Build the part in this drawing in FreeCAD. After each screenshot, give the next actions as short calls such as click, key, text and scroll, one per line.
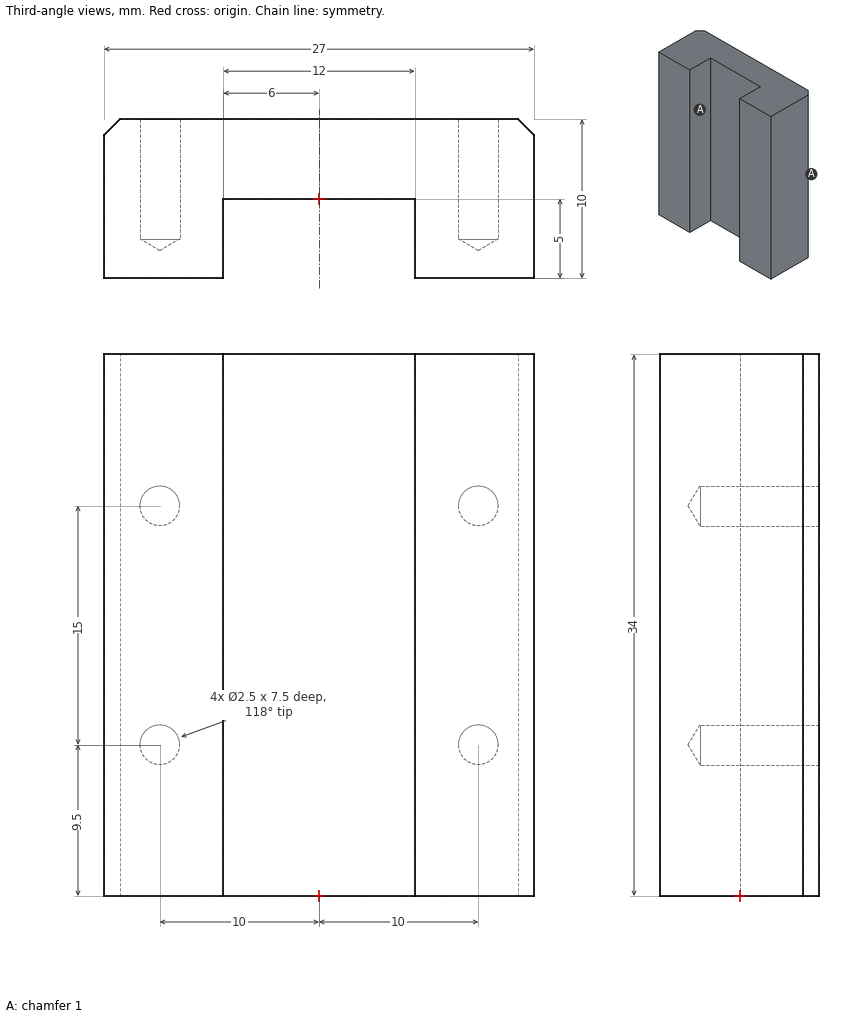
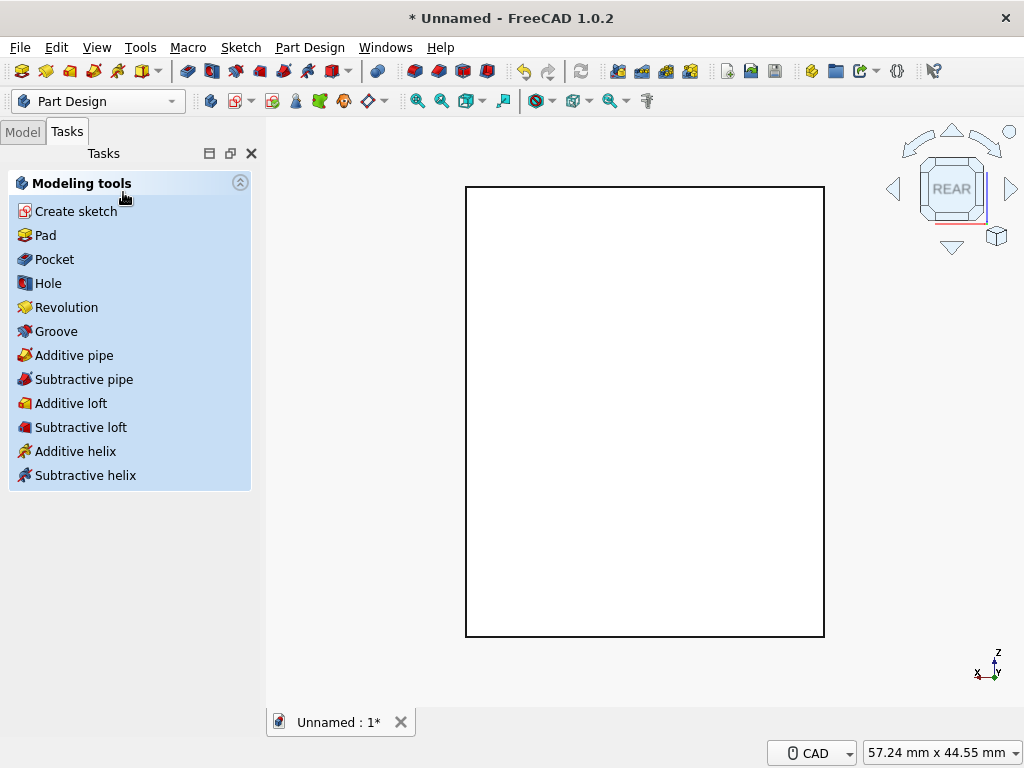
click(212, 72)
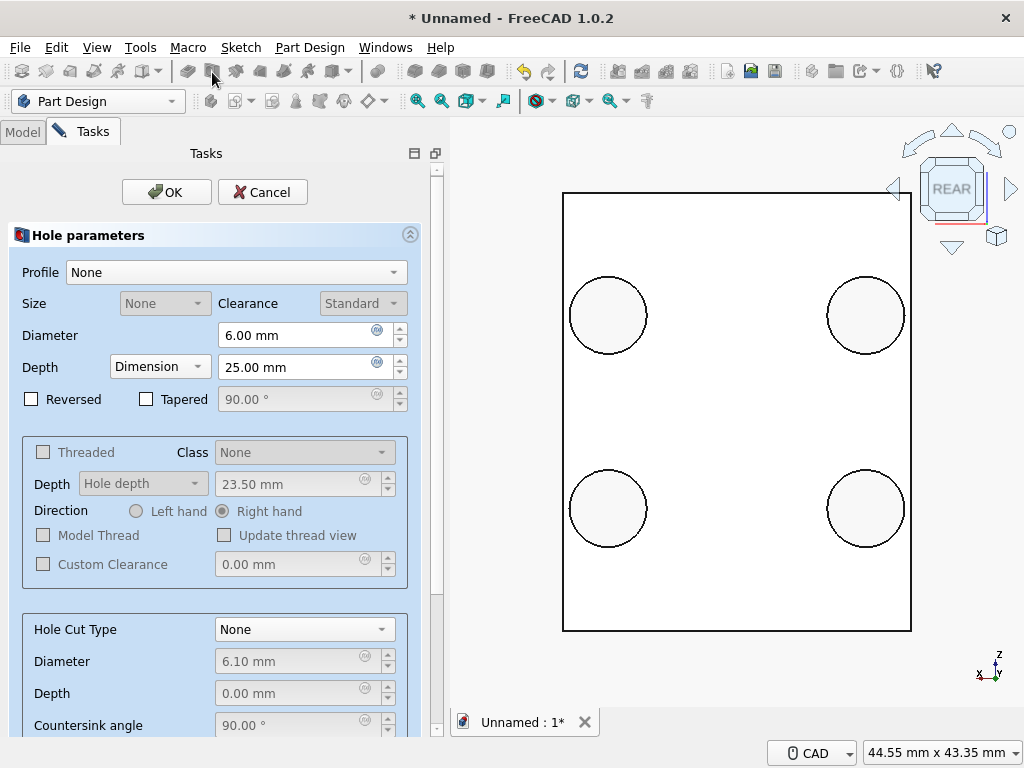
triple_click(305, 335)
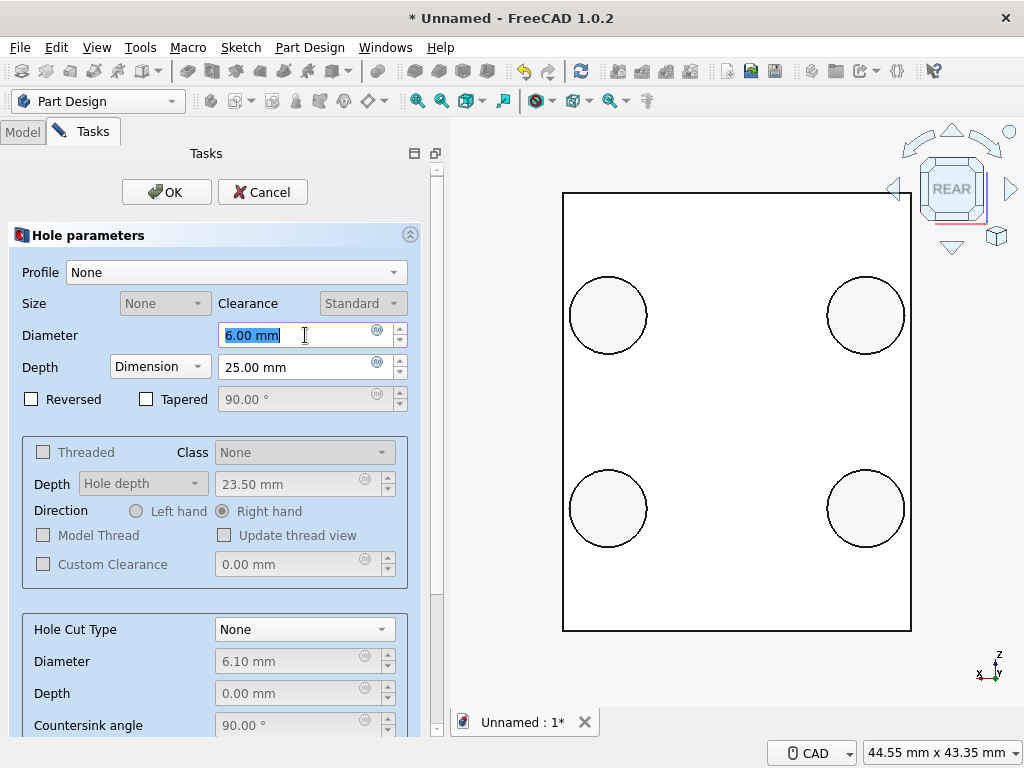
text(2.5)
key(Tab)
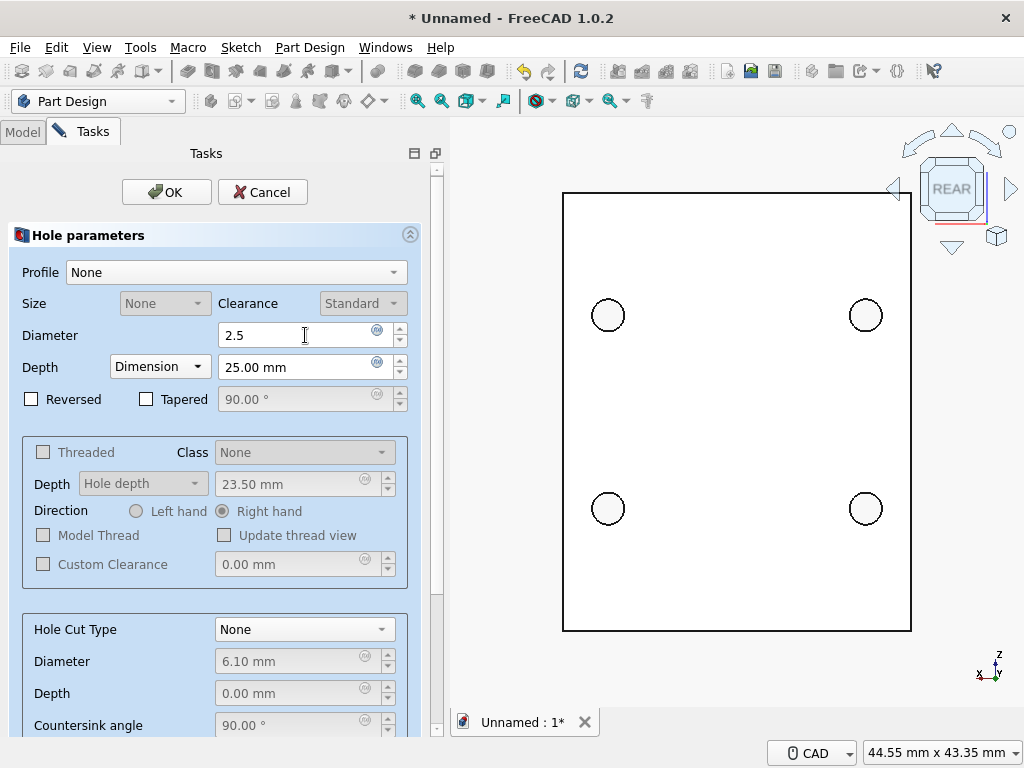
triple_click(305, 367)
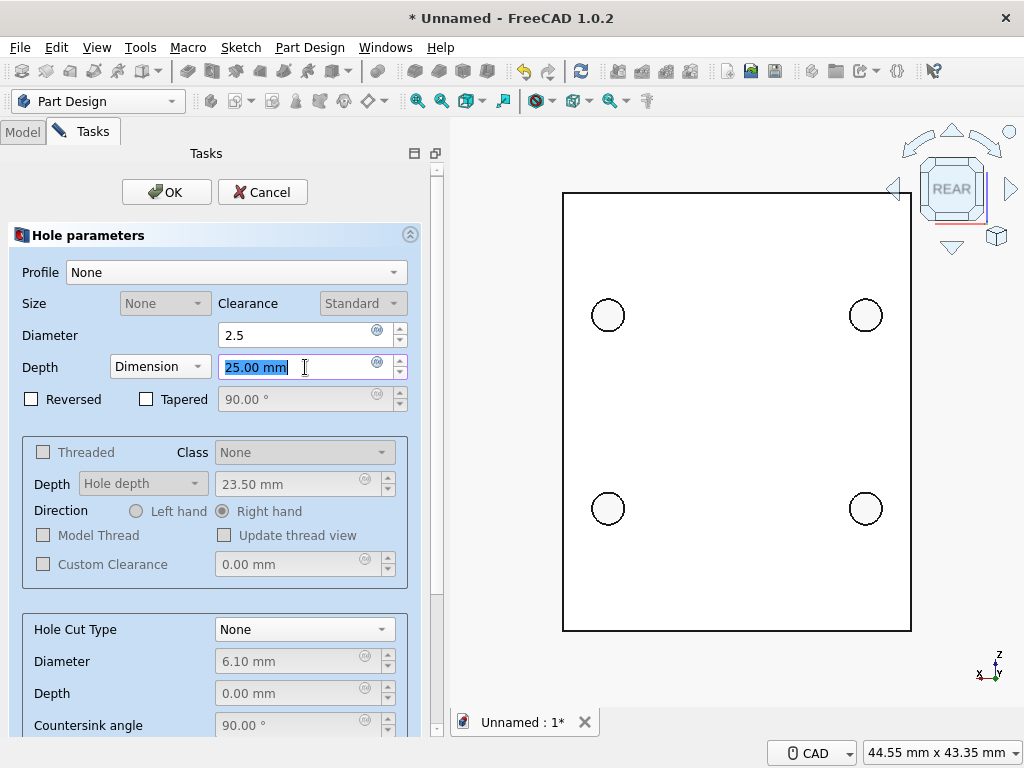
text(7.5)
key(Tab)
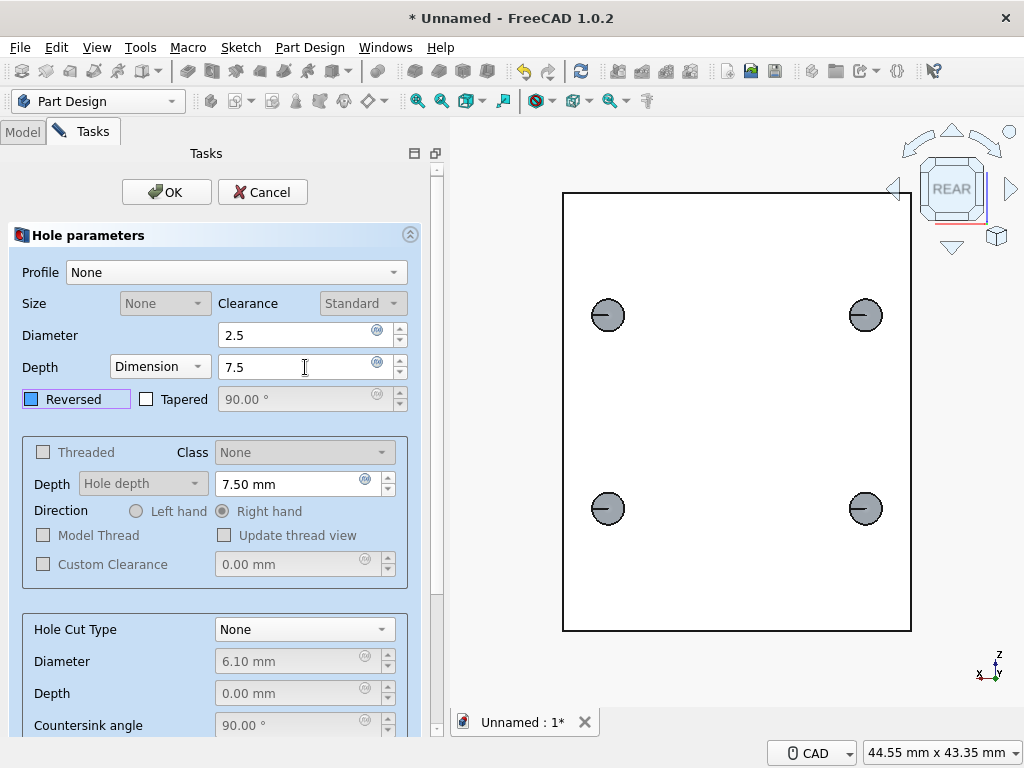
click(167, 192)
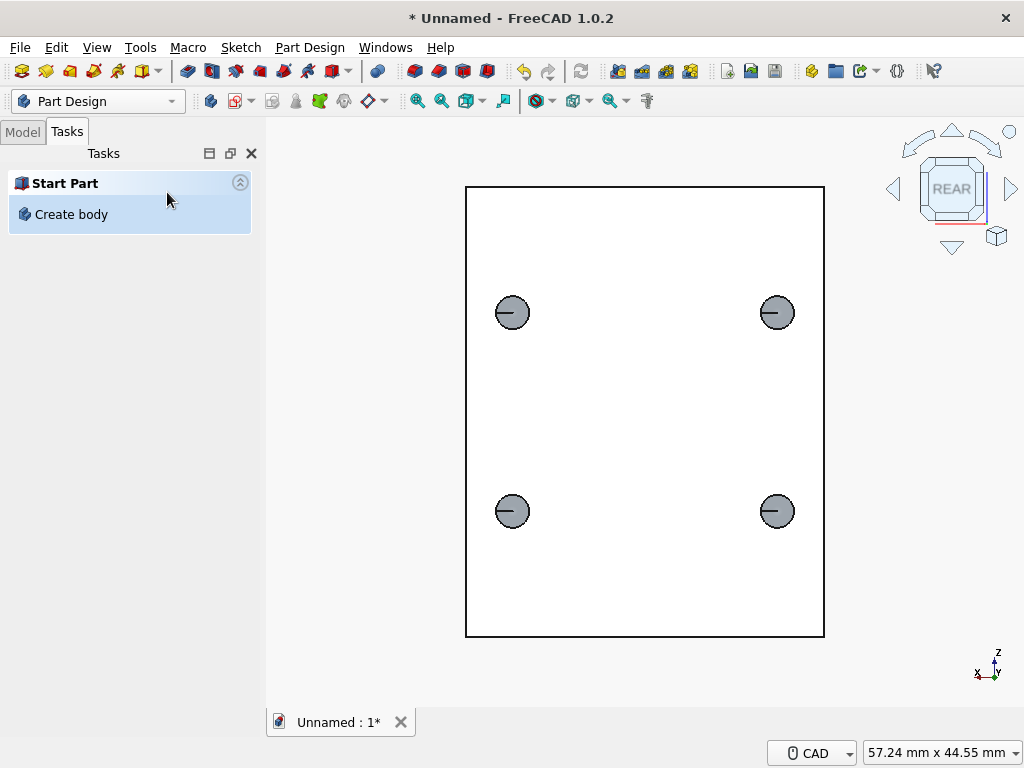
click(824, 411)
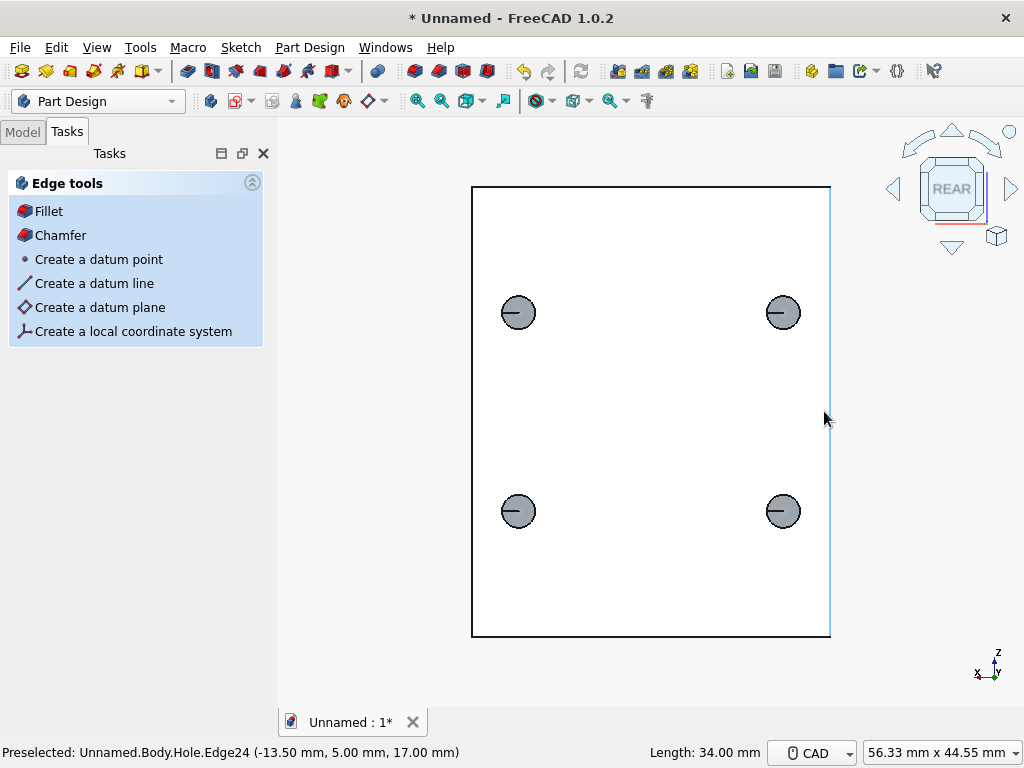
key(0)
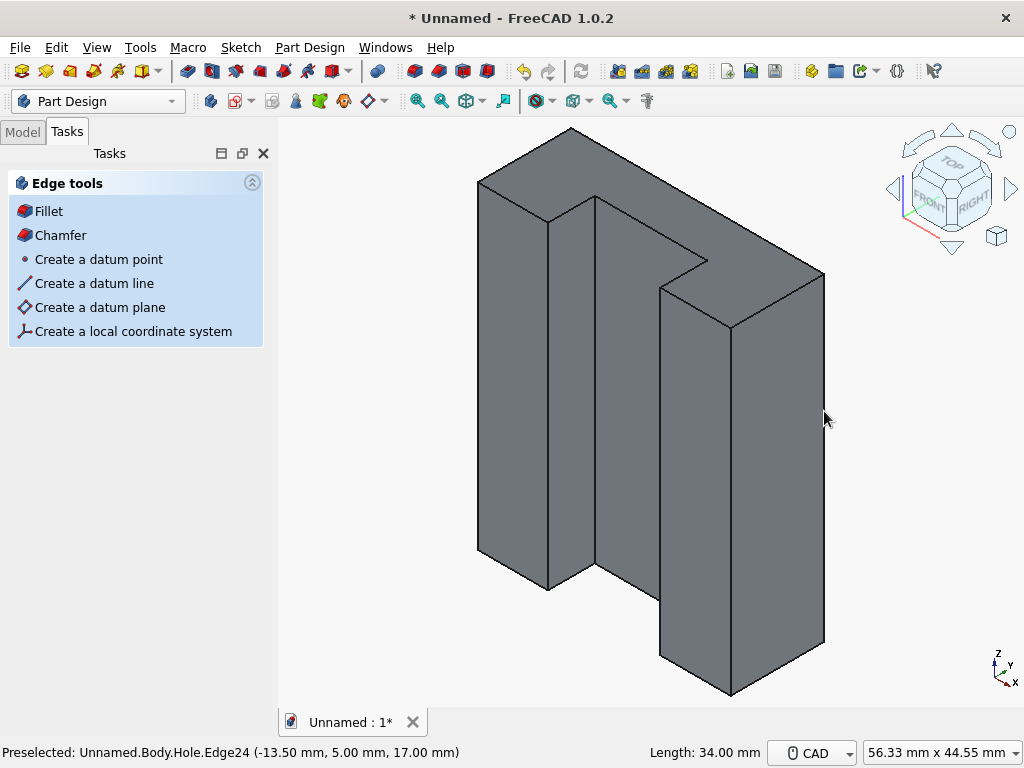
key(2)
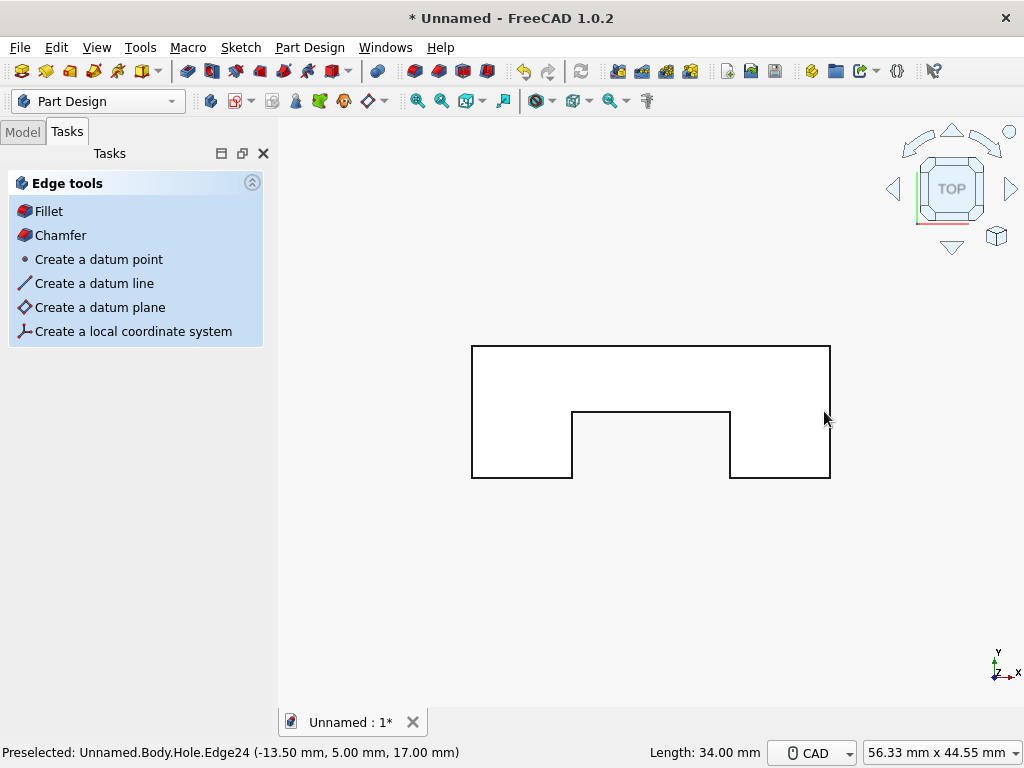
key(1)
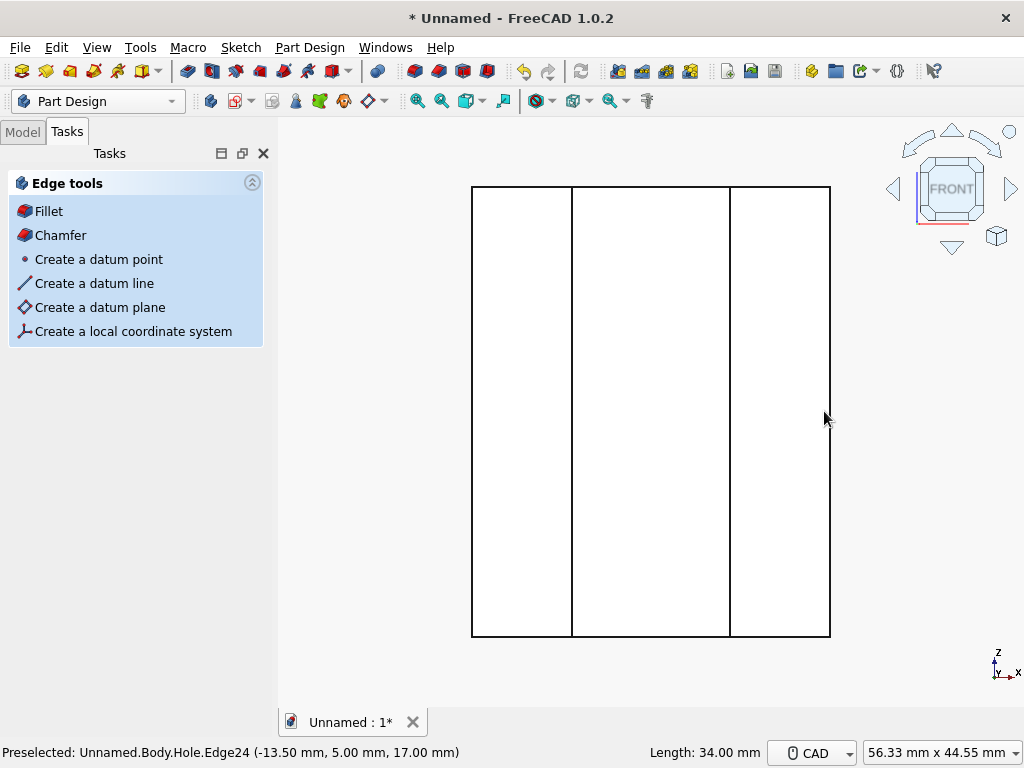
key(3)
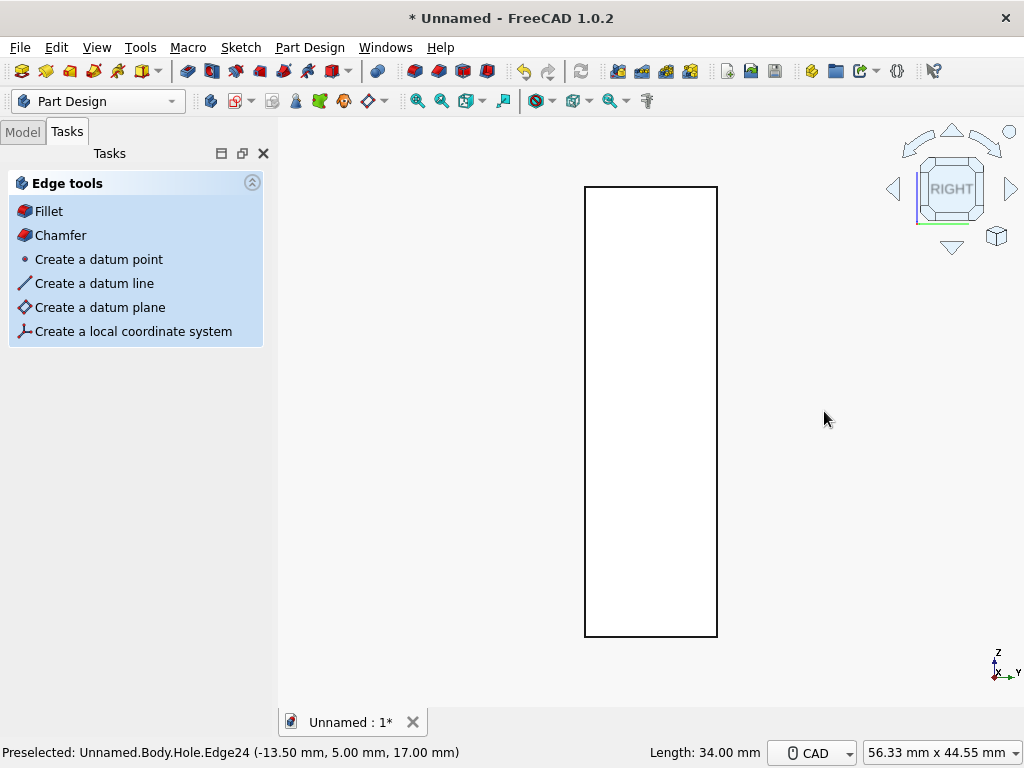
click(717, 411, ctrl)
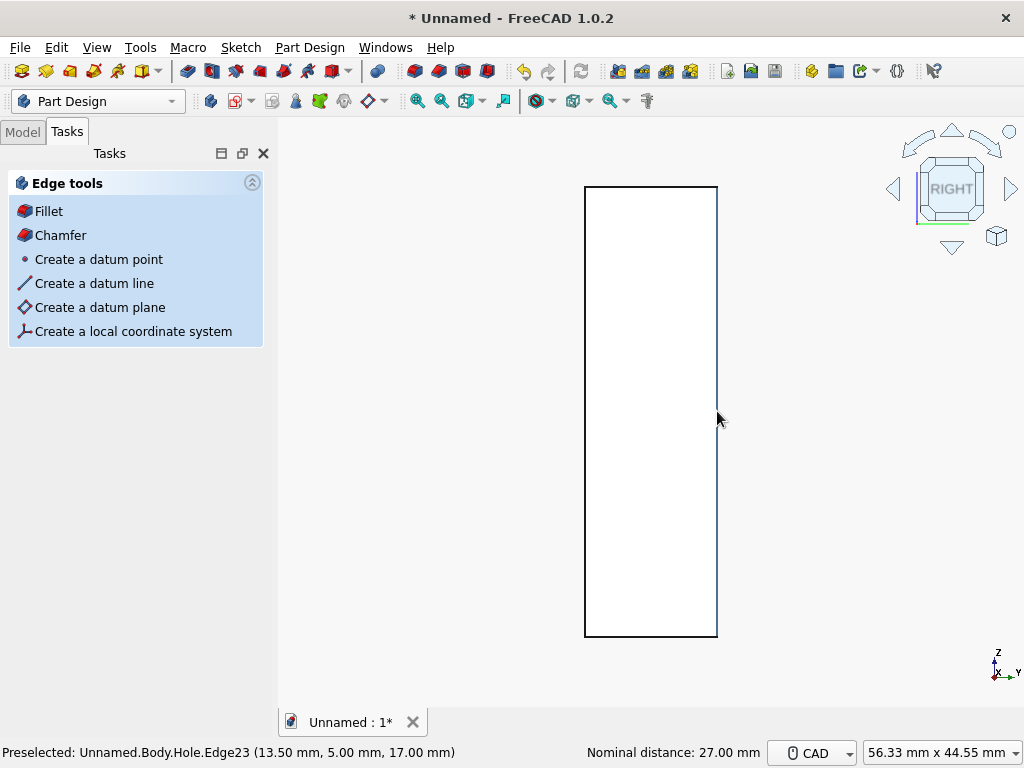
click(440, 72)